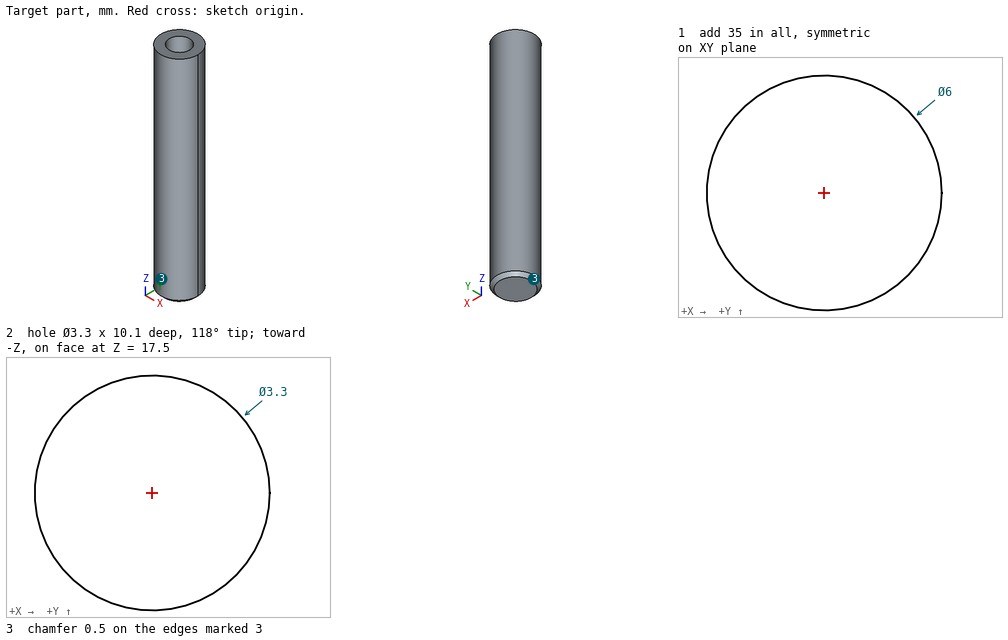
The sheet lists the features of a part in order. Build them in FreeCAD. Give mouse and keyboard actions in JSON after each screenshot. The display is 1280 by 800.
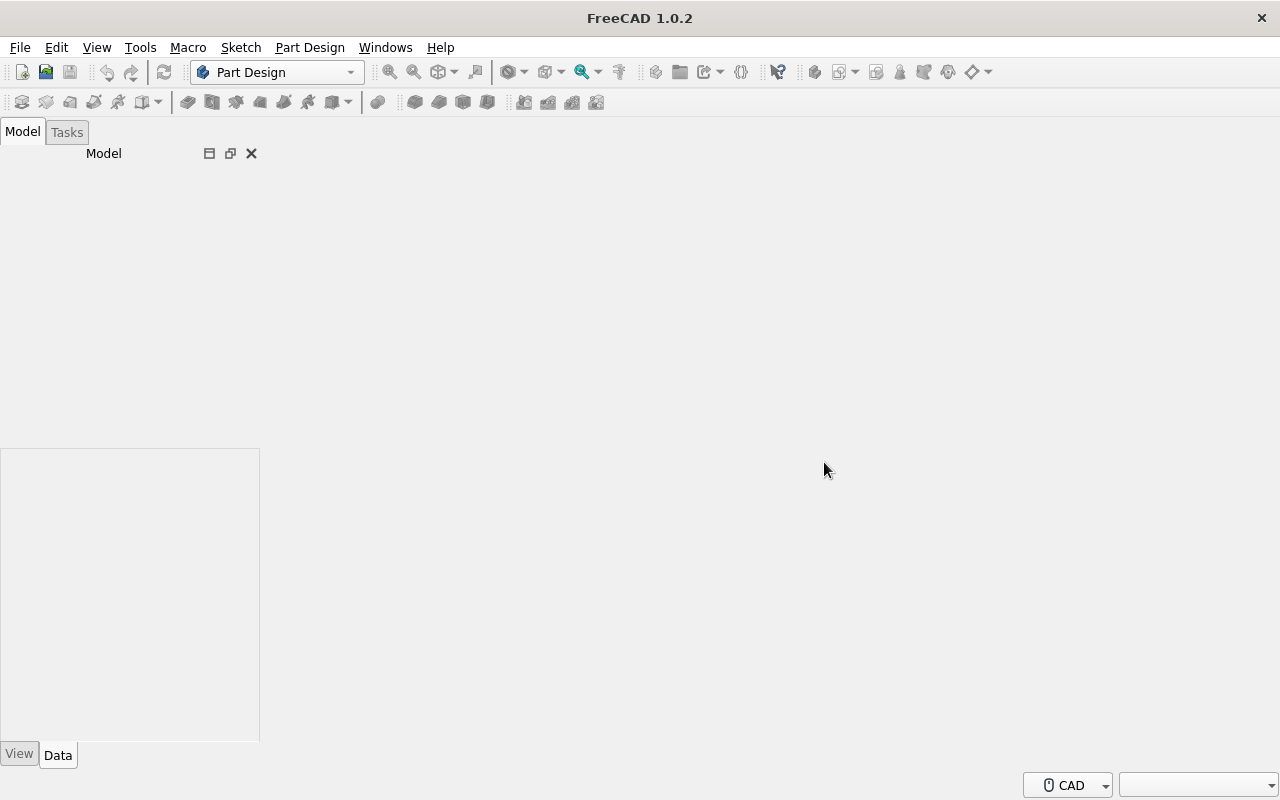
{"action": "left_click", "coordinate": [22, 72]}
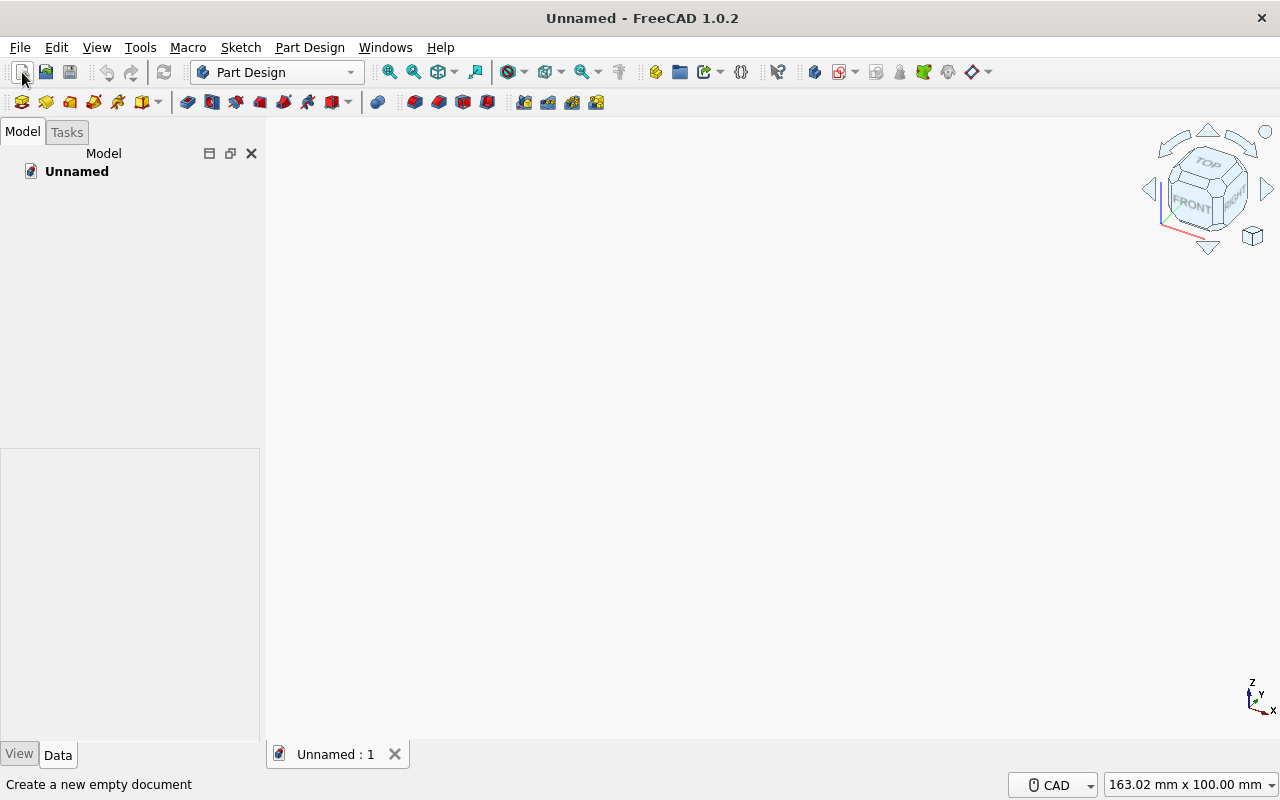
{"action": "left_click", "coordinate": [840, 72]}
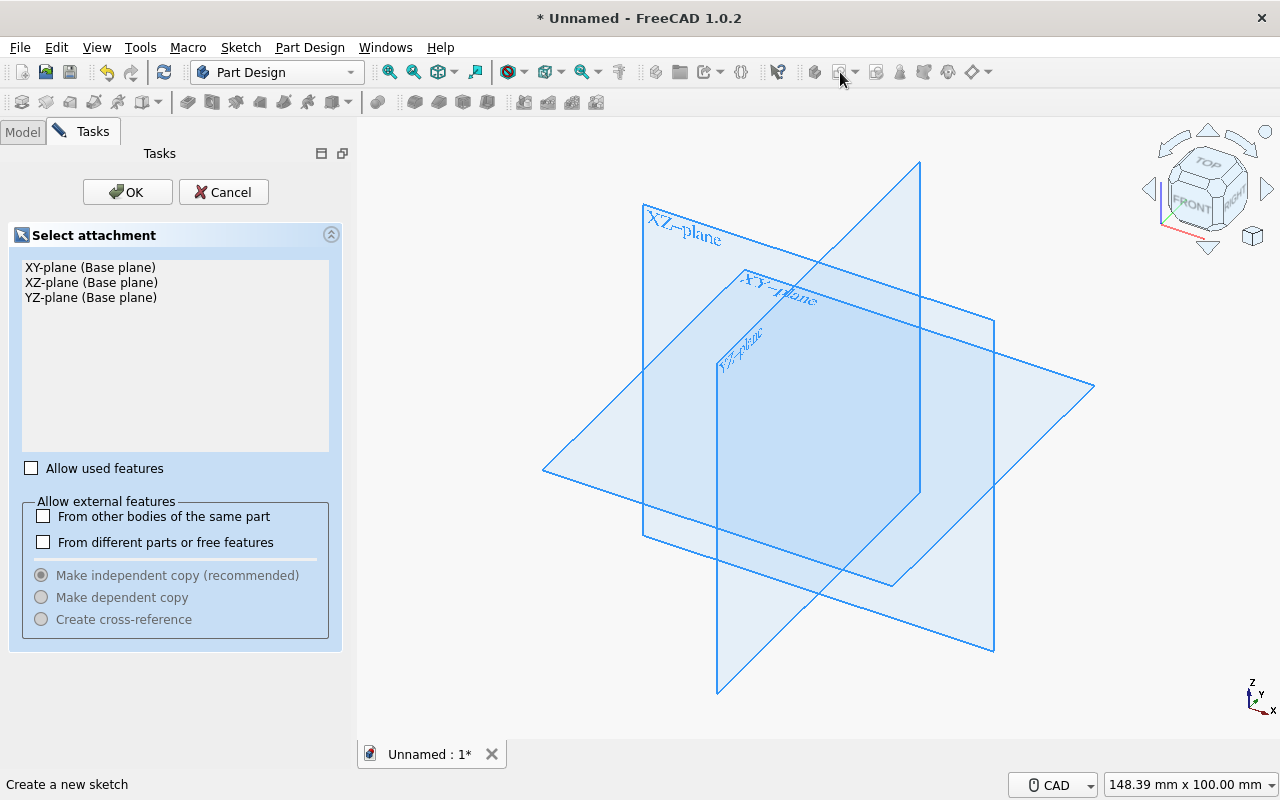
{"action": "left_click", "coordinate": [82, 268]}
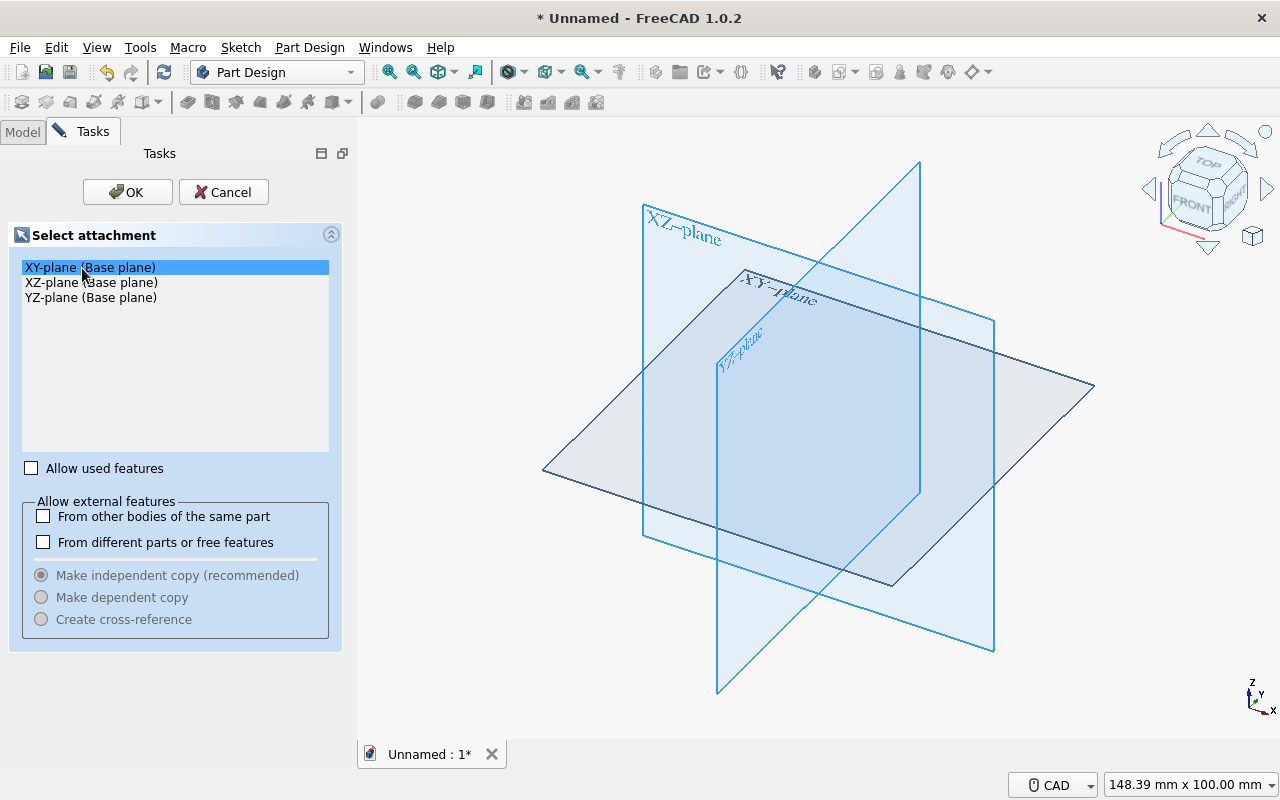
{"action": "left_click", "coordinate": [128, 192]}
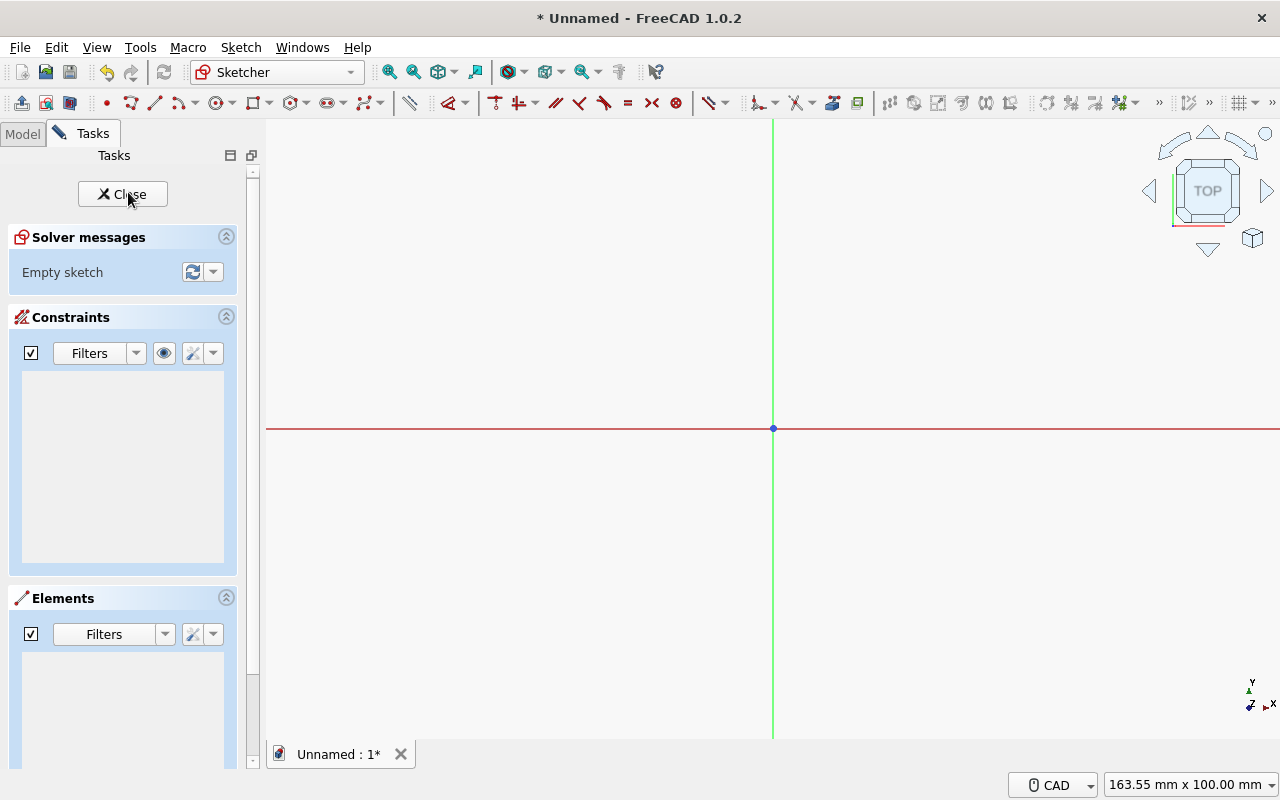
{"action": "scroll", "coordinate": [780, 429], "scroll_direction": "up", "scroll_amount": 12}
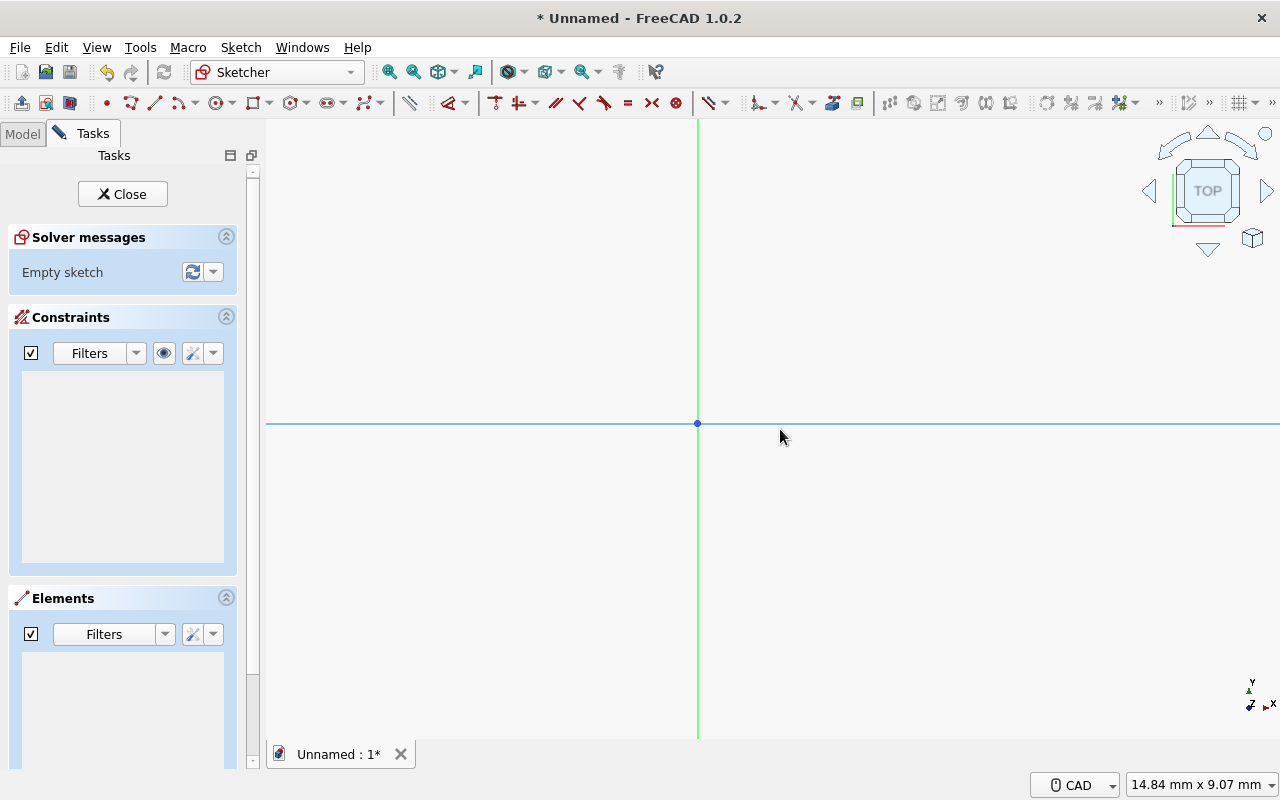
{"action": "left_click", "coordinate": [216, 104]}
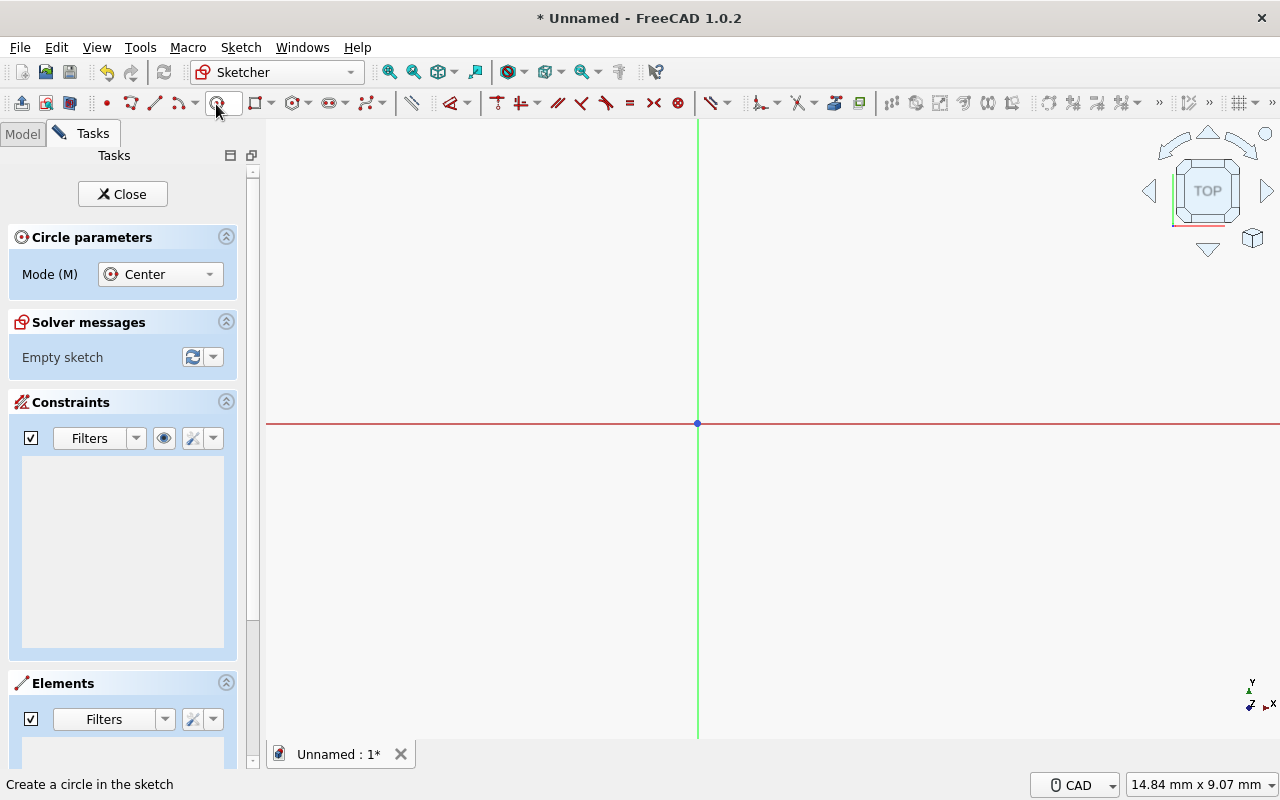
{"action": "left_click", "coordinate": [698, 424]}
{"action": "mouse_move", "coordinate": [843, 279]}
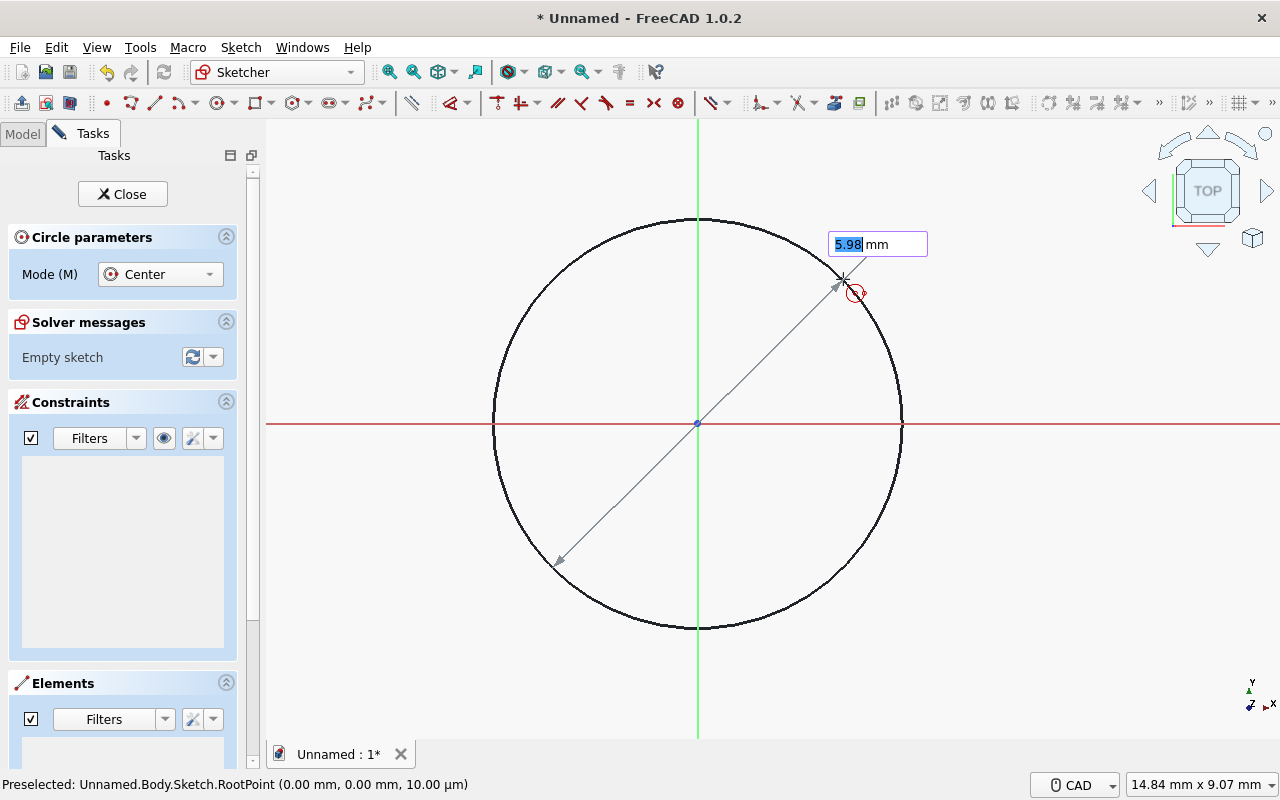
{"action": "type", "text": "6"}
{"action": "key", "text": "Return"}
{"action": "key", "text": "Escape"}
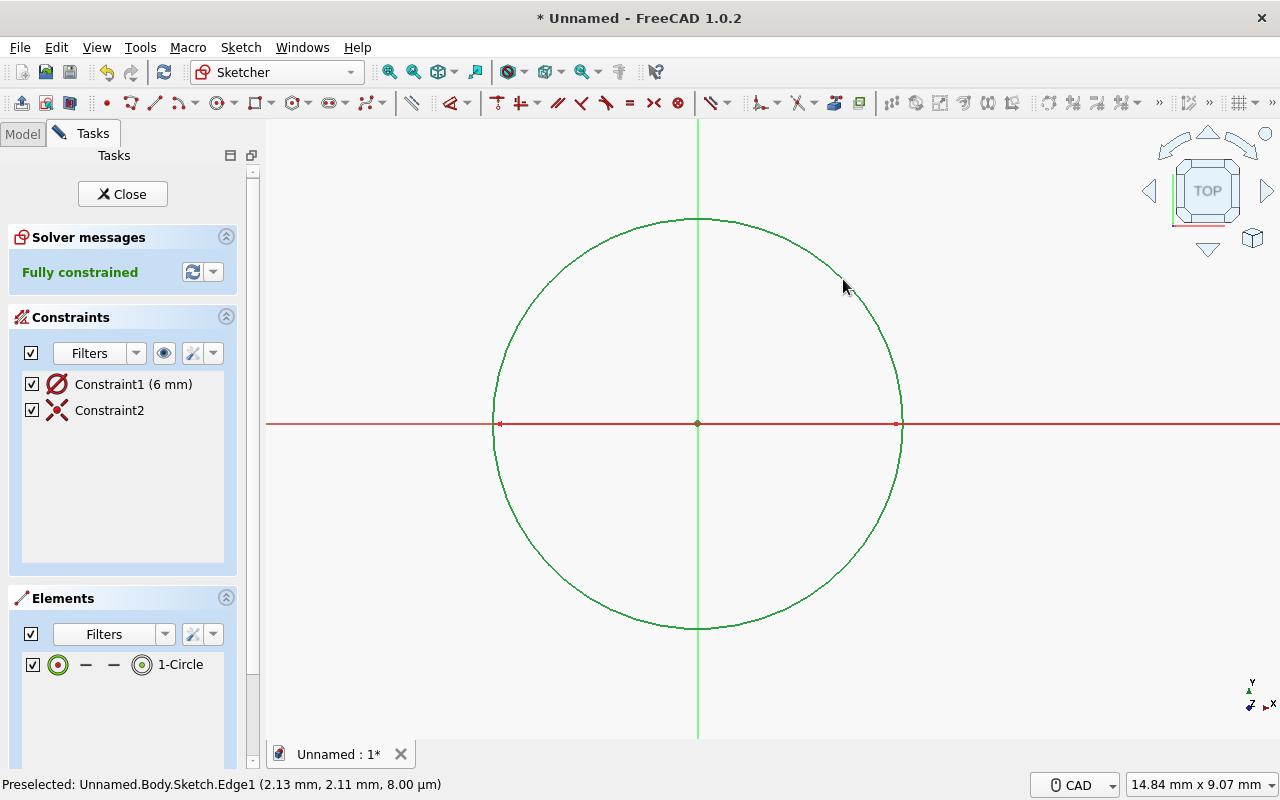
{"action": "left_click", "coordinate": [123, 194]}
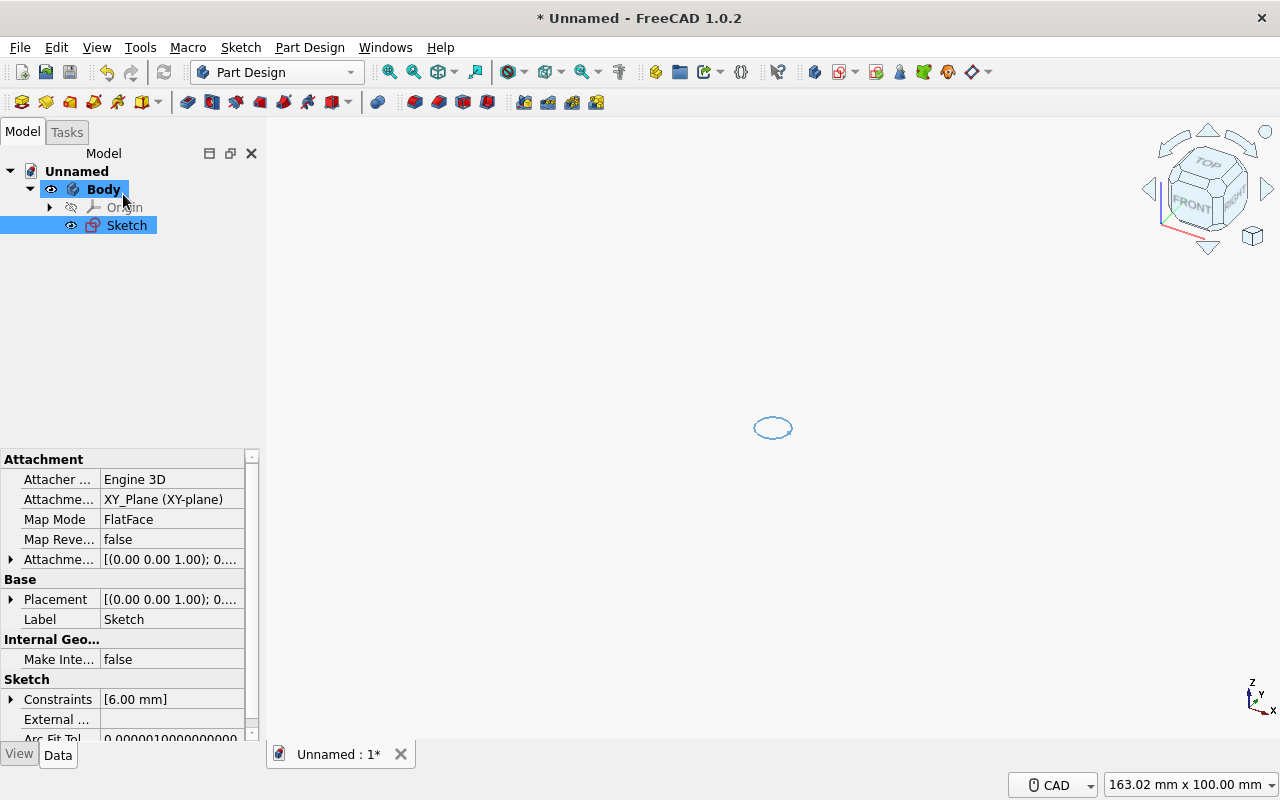
{"action": "left_click", "coordinate": [22, 102]}